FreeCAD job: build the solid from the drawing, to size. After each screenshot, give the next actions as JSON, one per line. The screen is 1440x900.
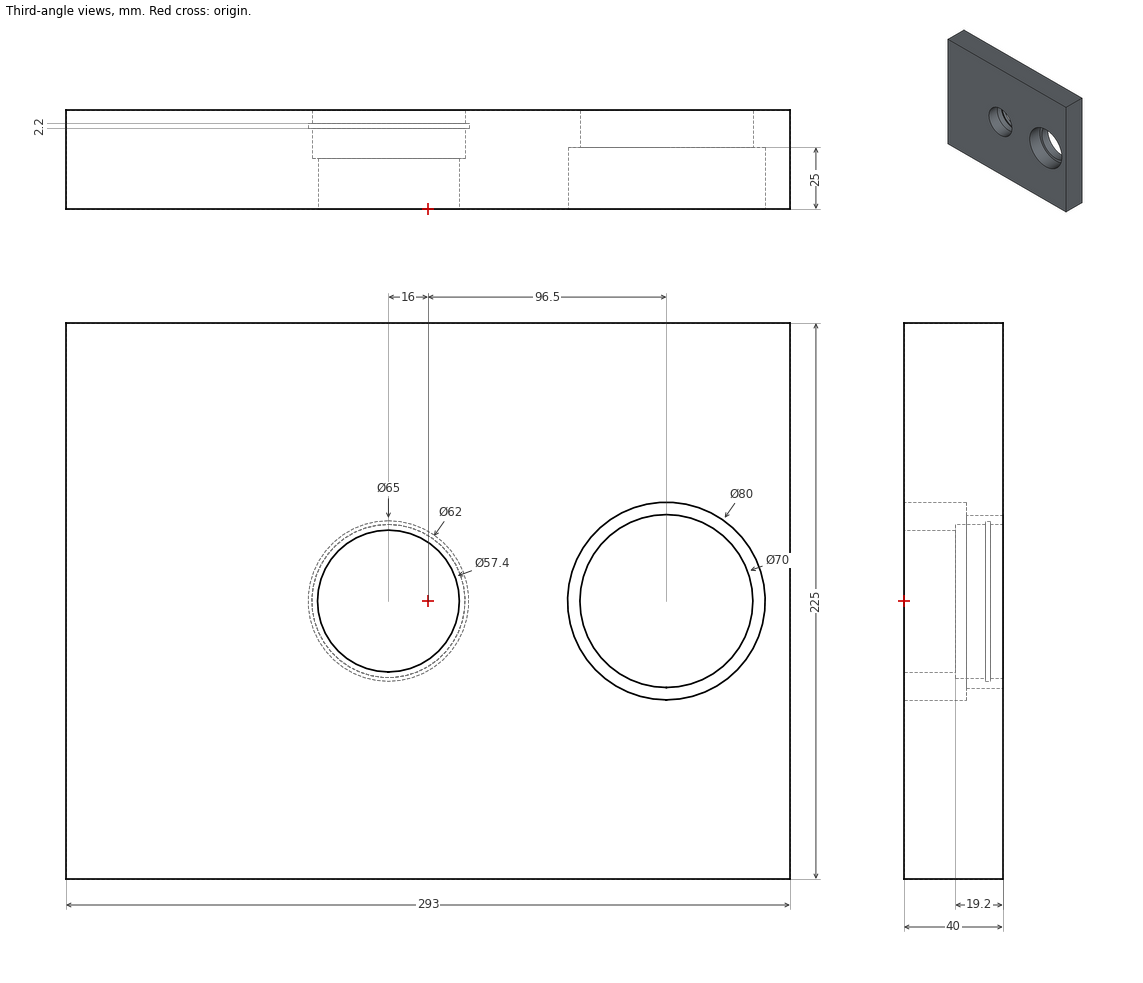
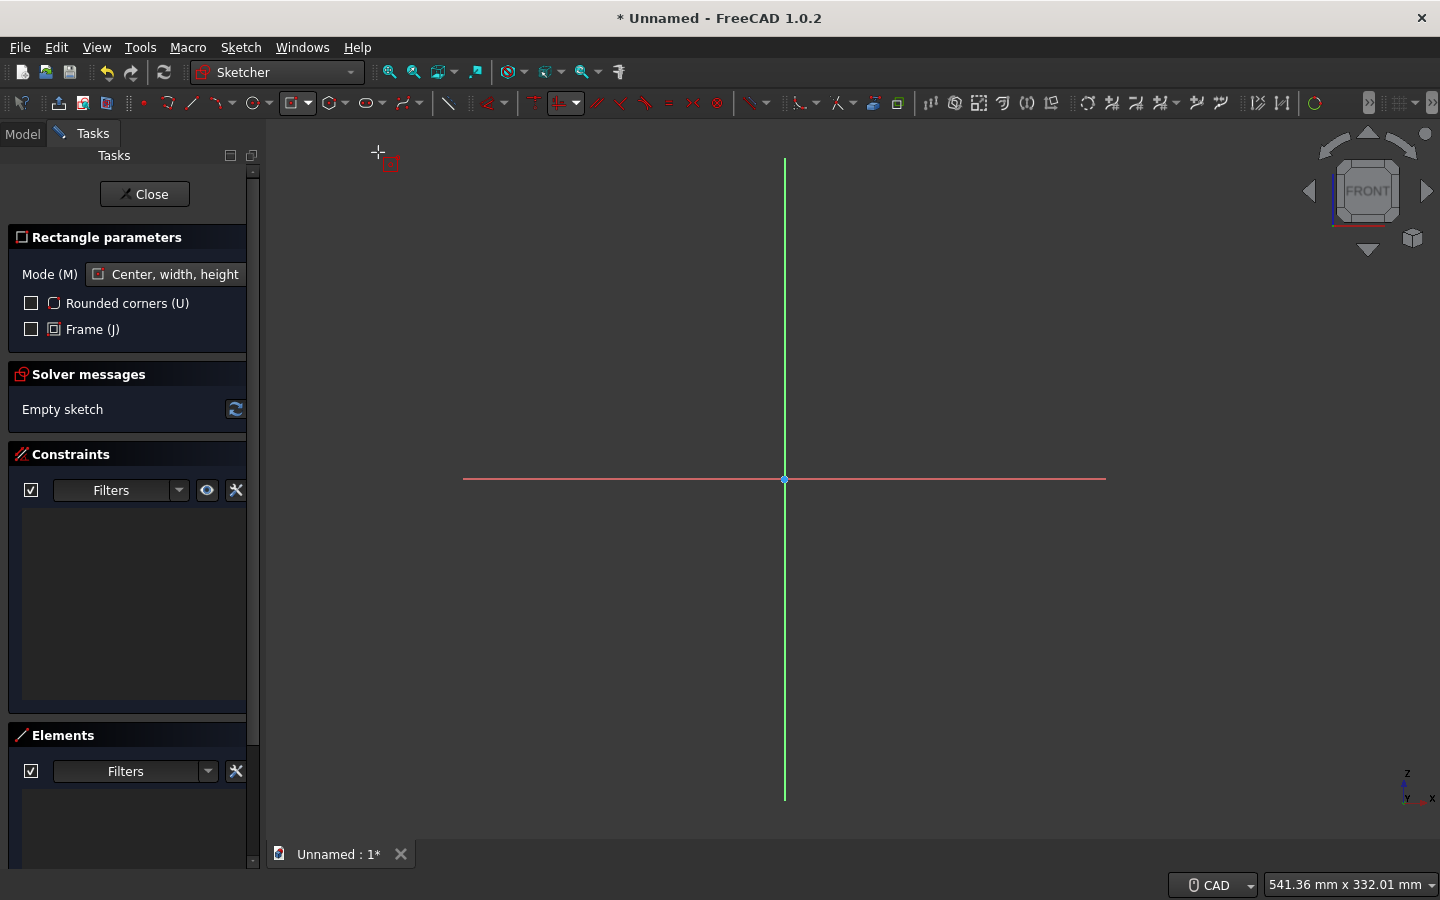
{"action": "left_click", "coordinate": [785, 479]}
{"action": "mouse_move", "coordinate": [1103, 235]}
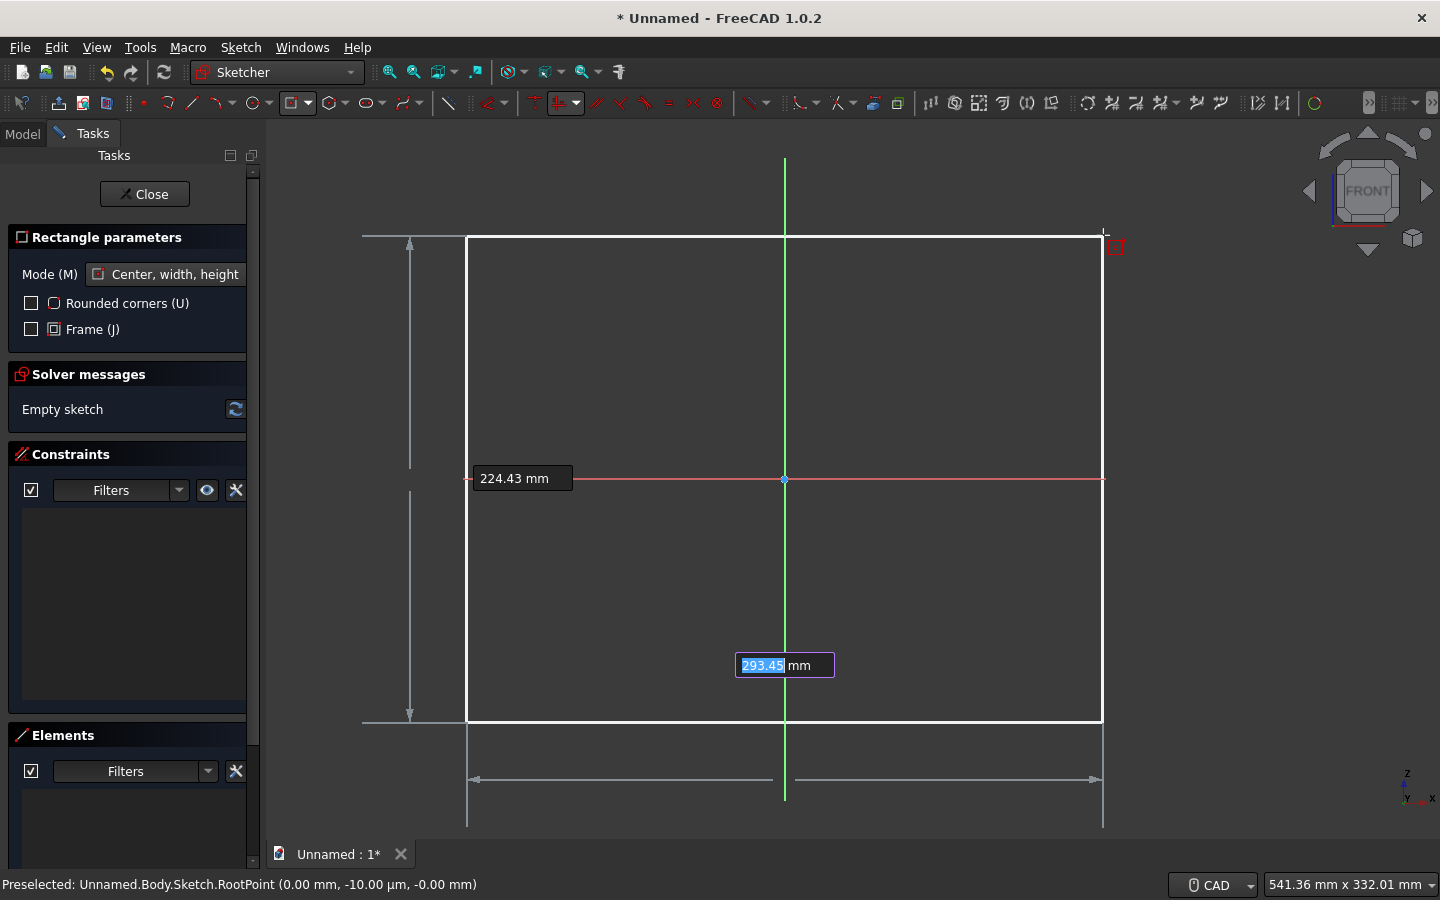
{"action": "type", "text": "293"}
{"action": "key", "text": "Tab"}
{"action": "type", "text": "225"}
{"action": "key", "text": "Return"}
{"action": "key", "text": "Escape"}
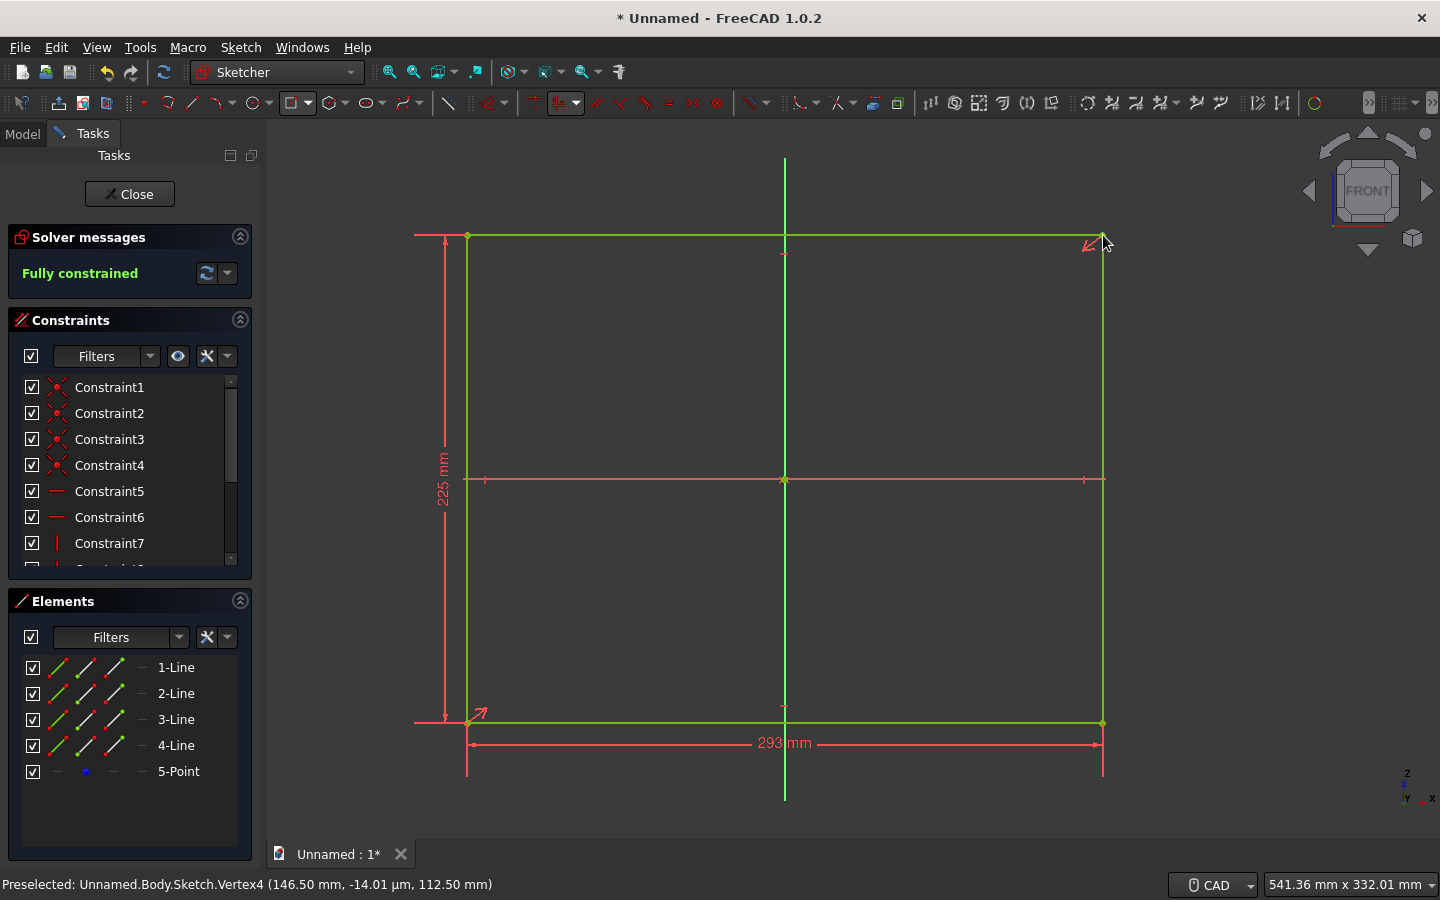
{"action": "left_click", "coordinate": [130, 194]}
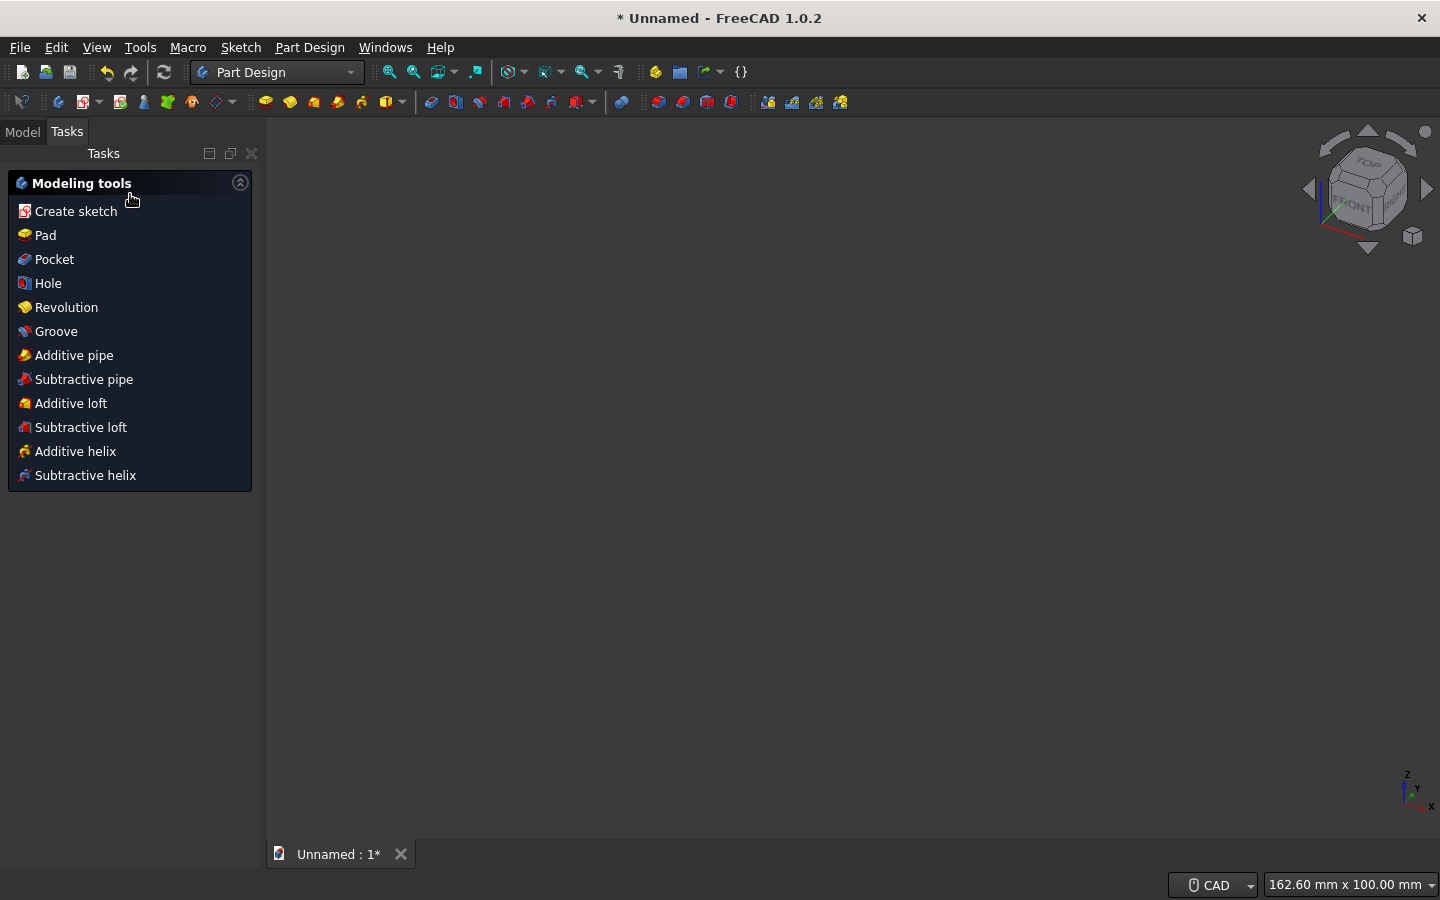
{"action": "left_click", "coordinate": [266, 102]}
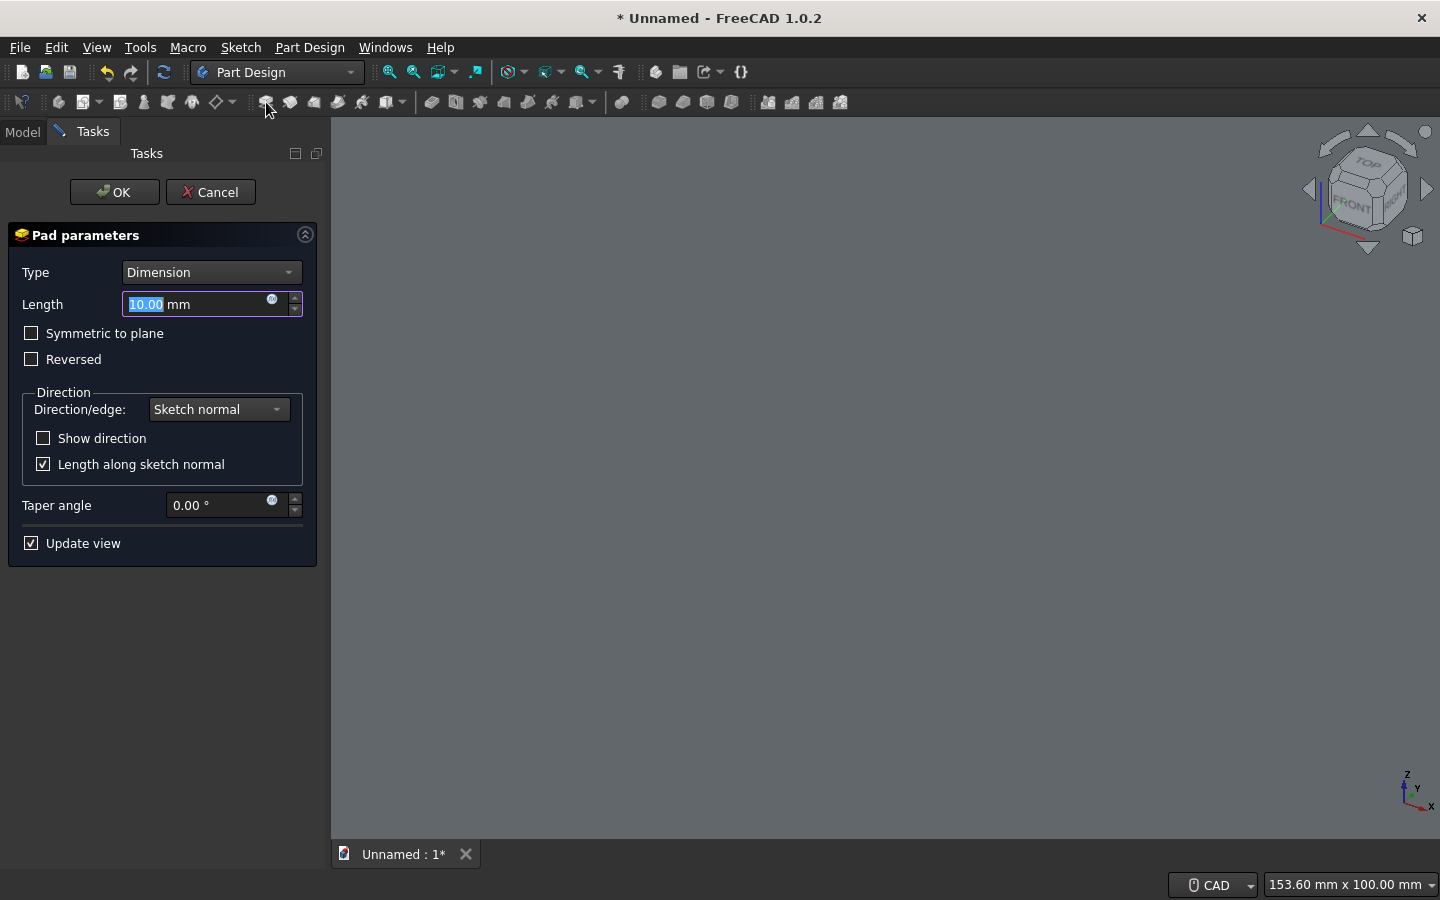
{"action": "type", "text": "40"}
{"action": "key", "text": "Tab"}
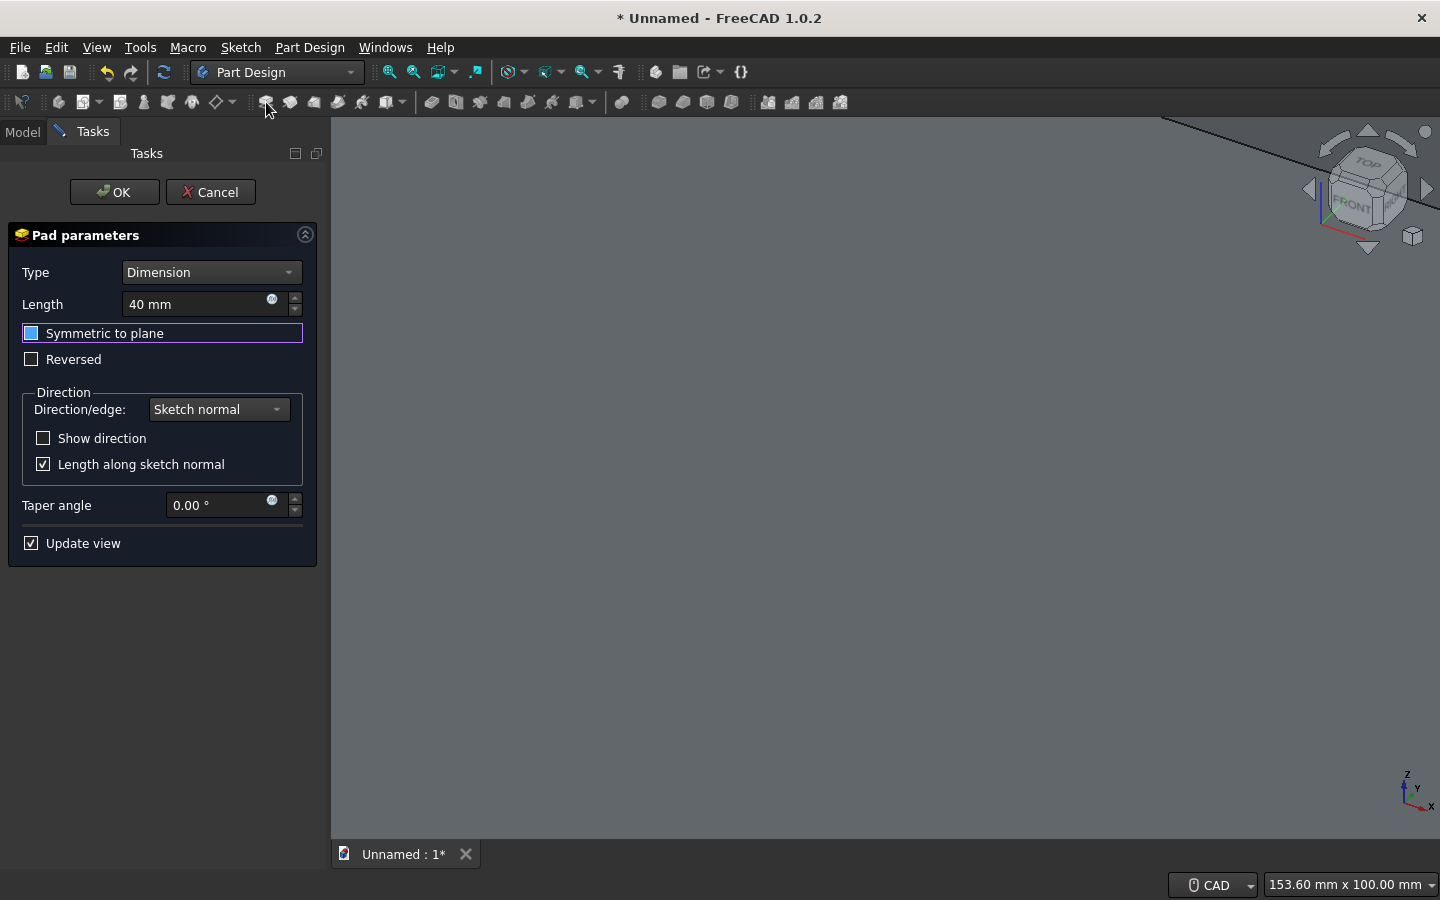
{"action": "left_click", "coordinate": [30, 359]}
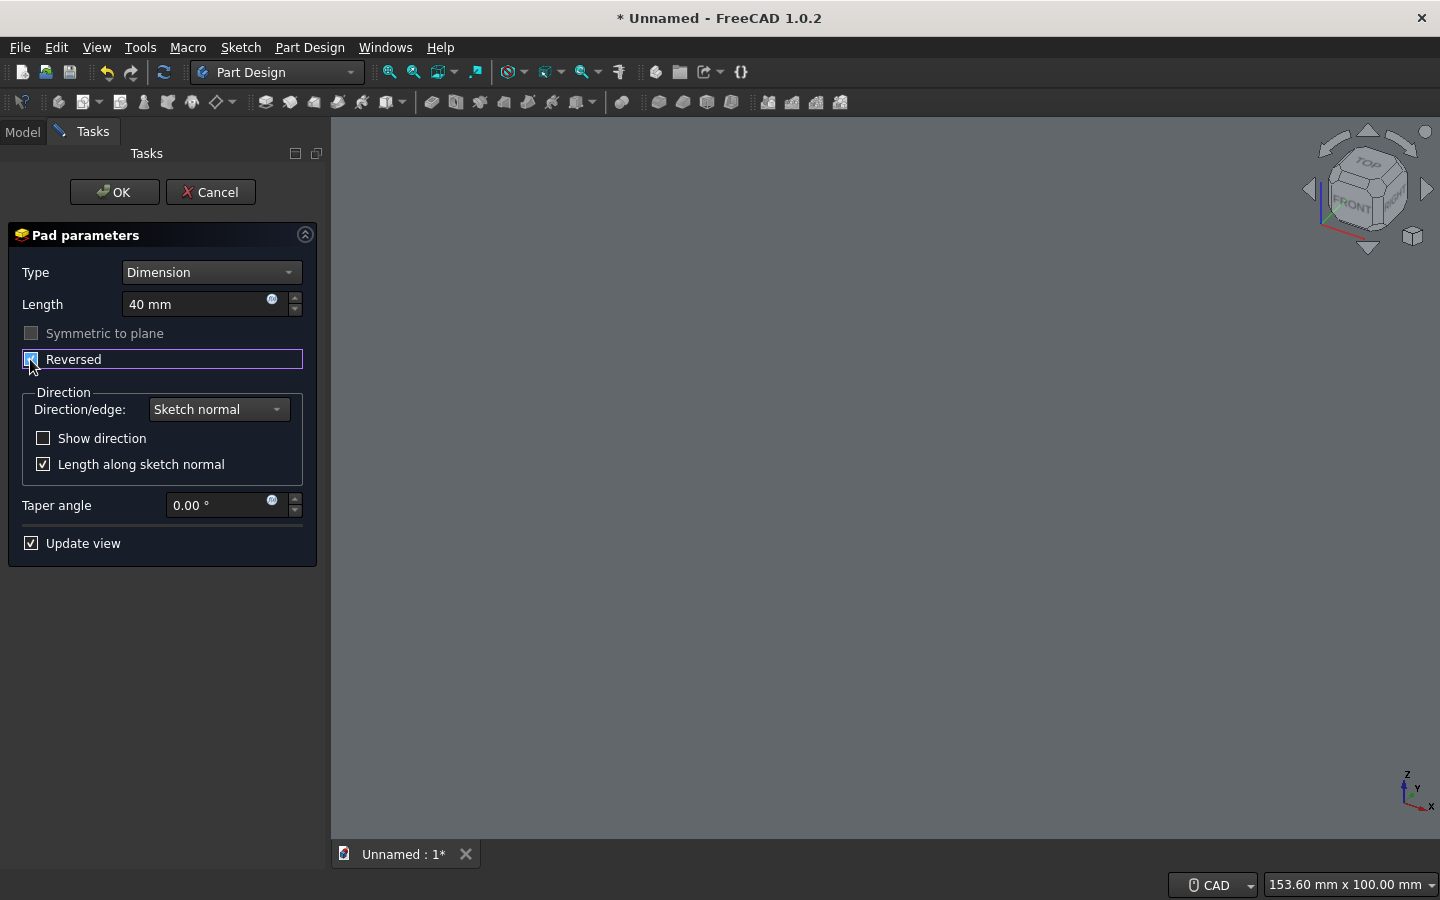
{"action": "left_click", "coordinate": [115, 192]}